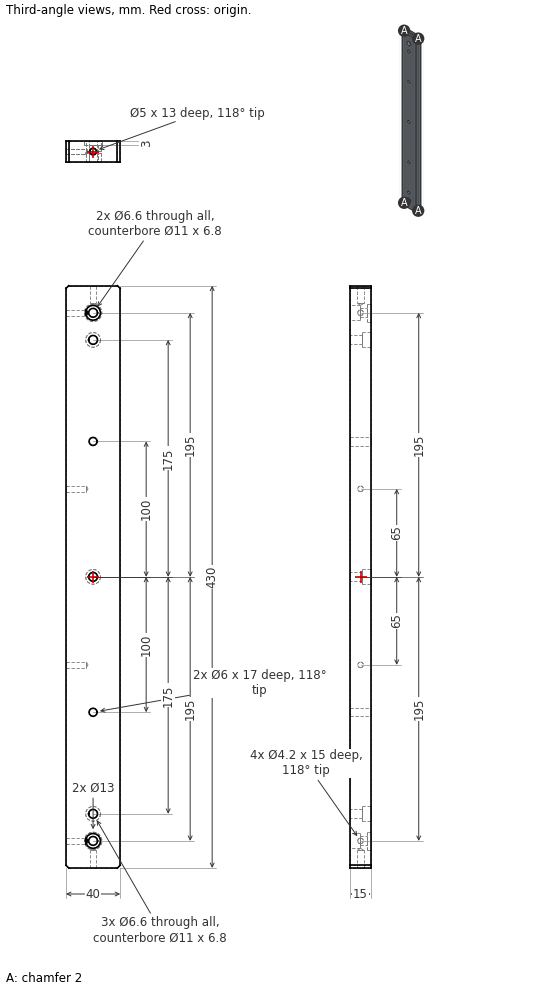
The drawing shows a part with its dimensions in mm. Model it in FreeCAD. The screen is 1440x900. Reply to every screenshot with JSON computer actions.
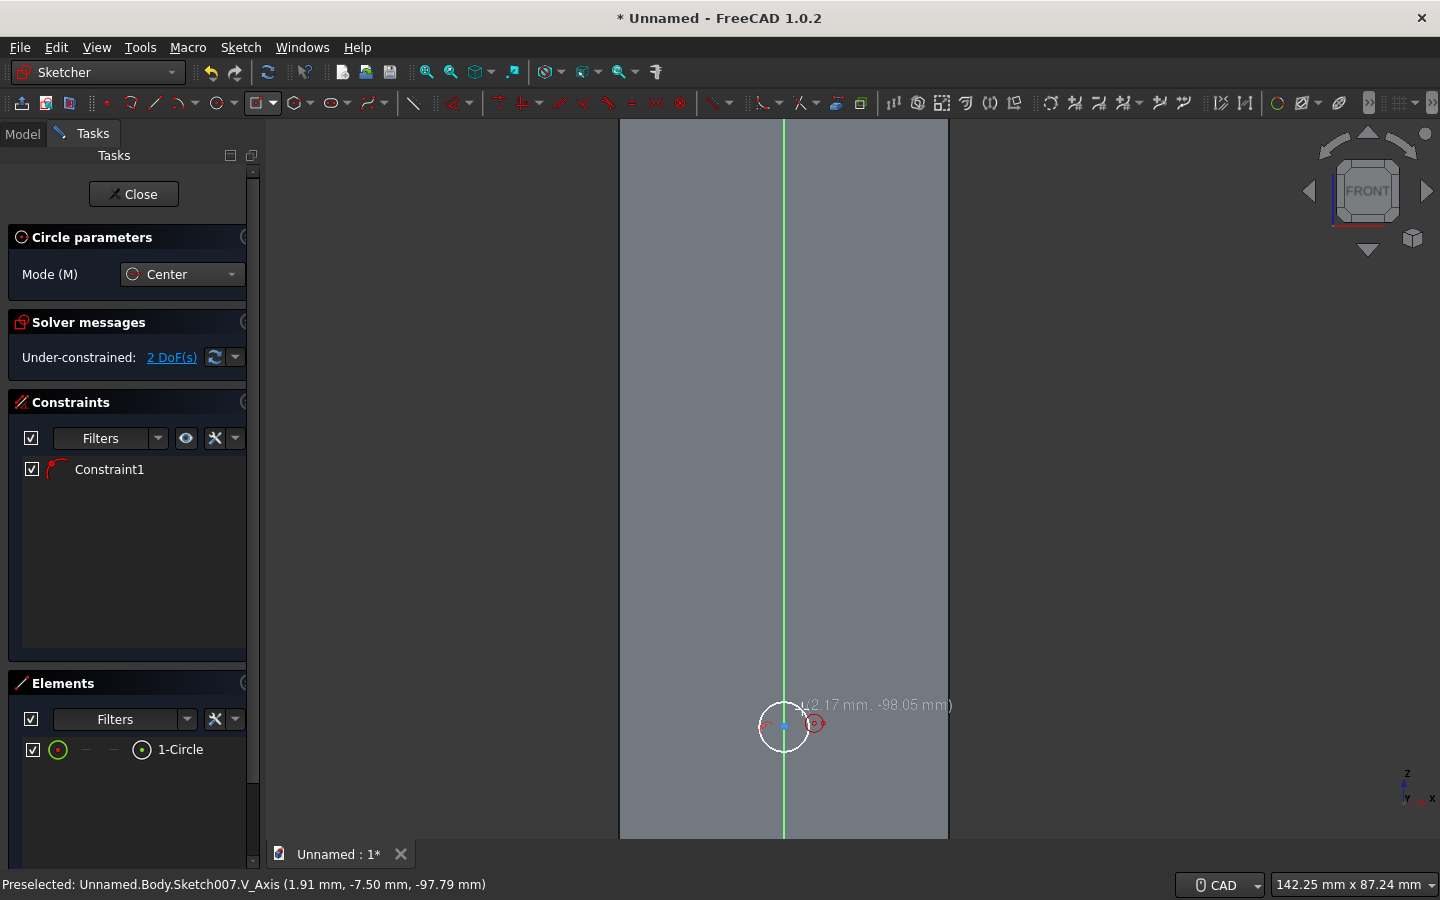
{"action": "scroll", "coordinate": [785, 728], "scroll_direction": "down", "scroll_amount": 6}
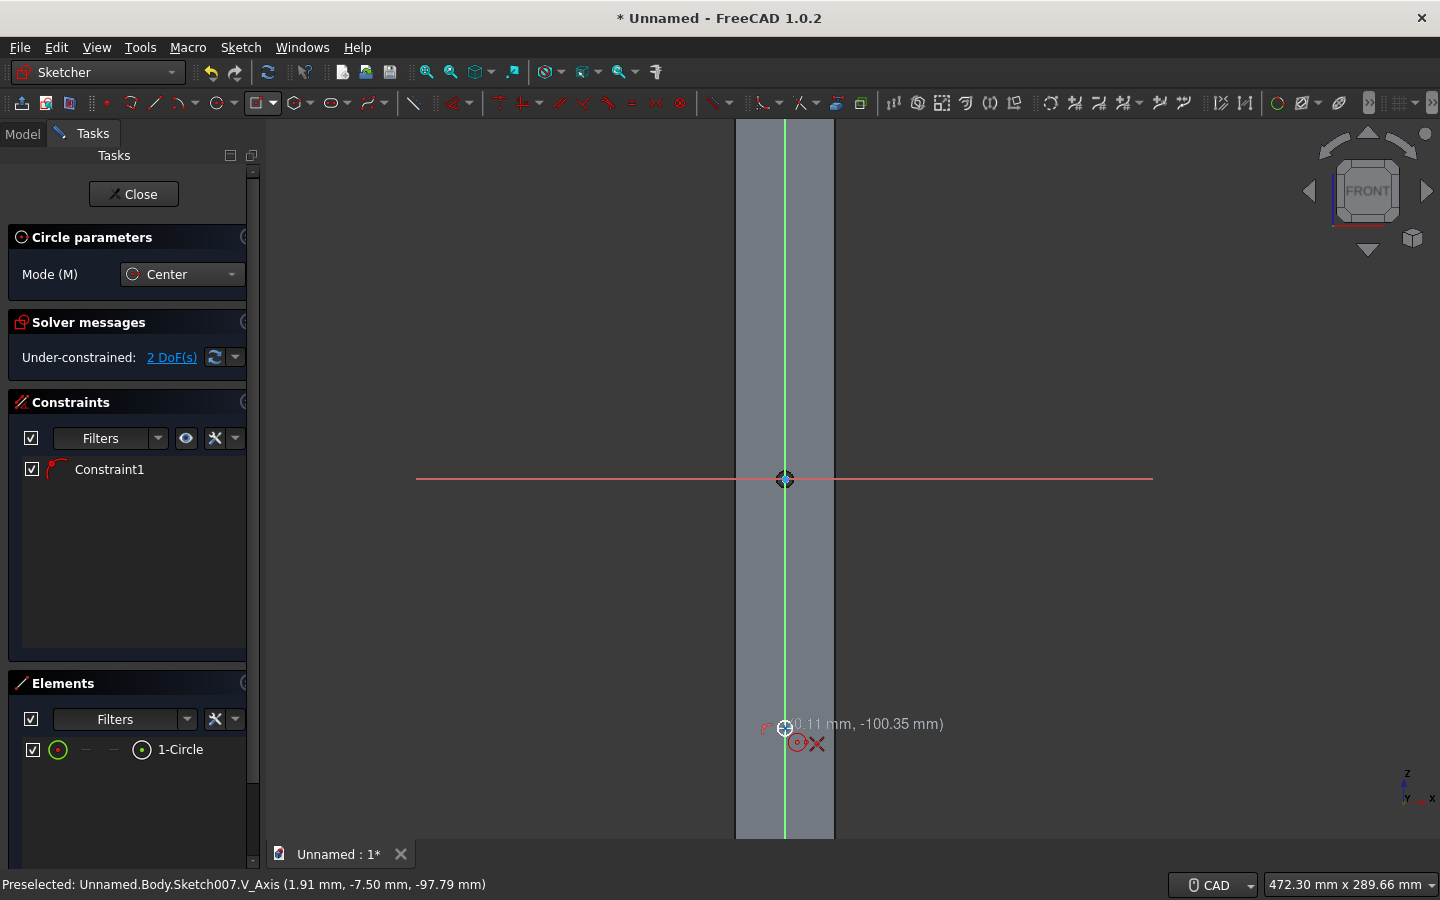
{"action": "scroll", "coordinate": [785, 231], "scroll_direction": "up", "scroll_amount": 6}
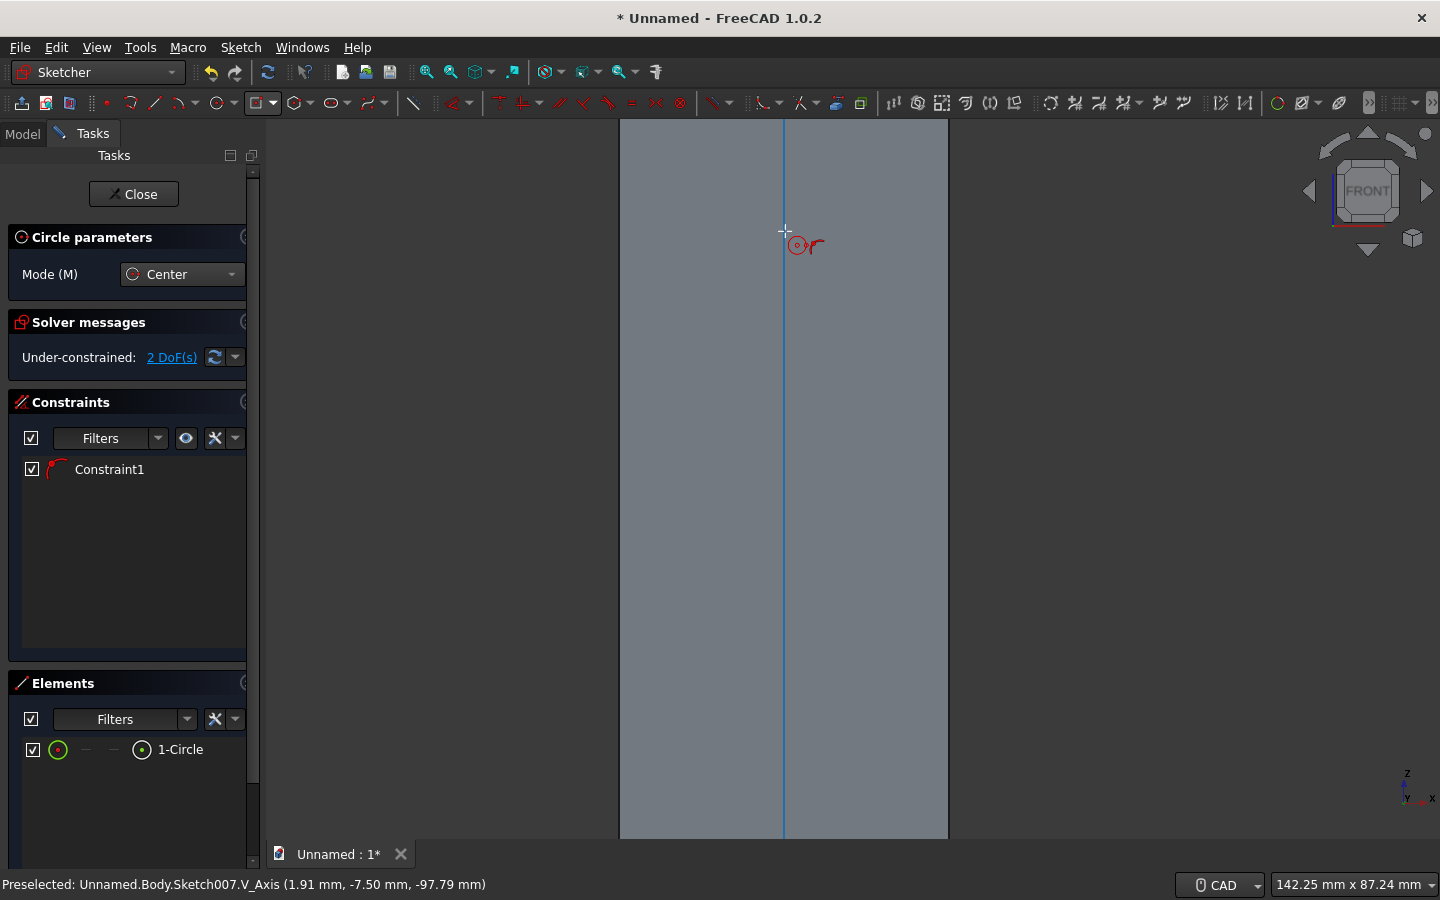
{"action": "left_click", "coordinate": [784, 230]}
{"action": "left_click", "coordinate": [802, 213]}
{"action": "key", "text": "Escape"}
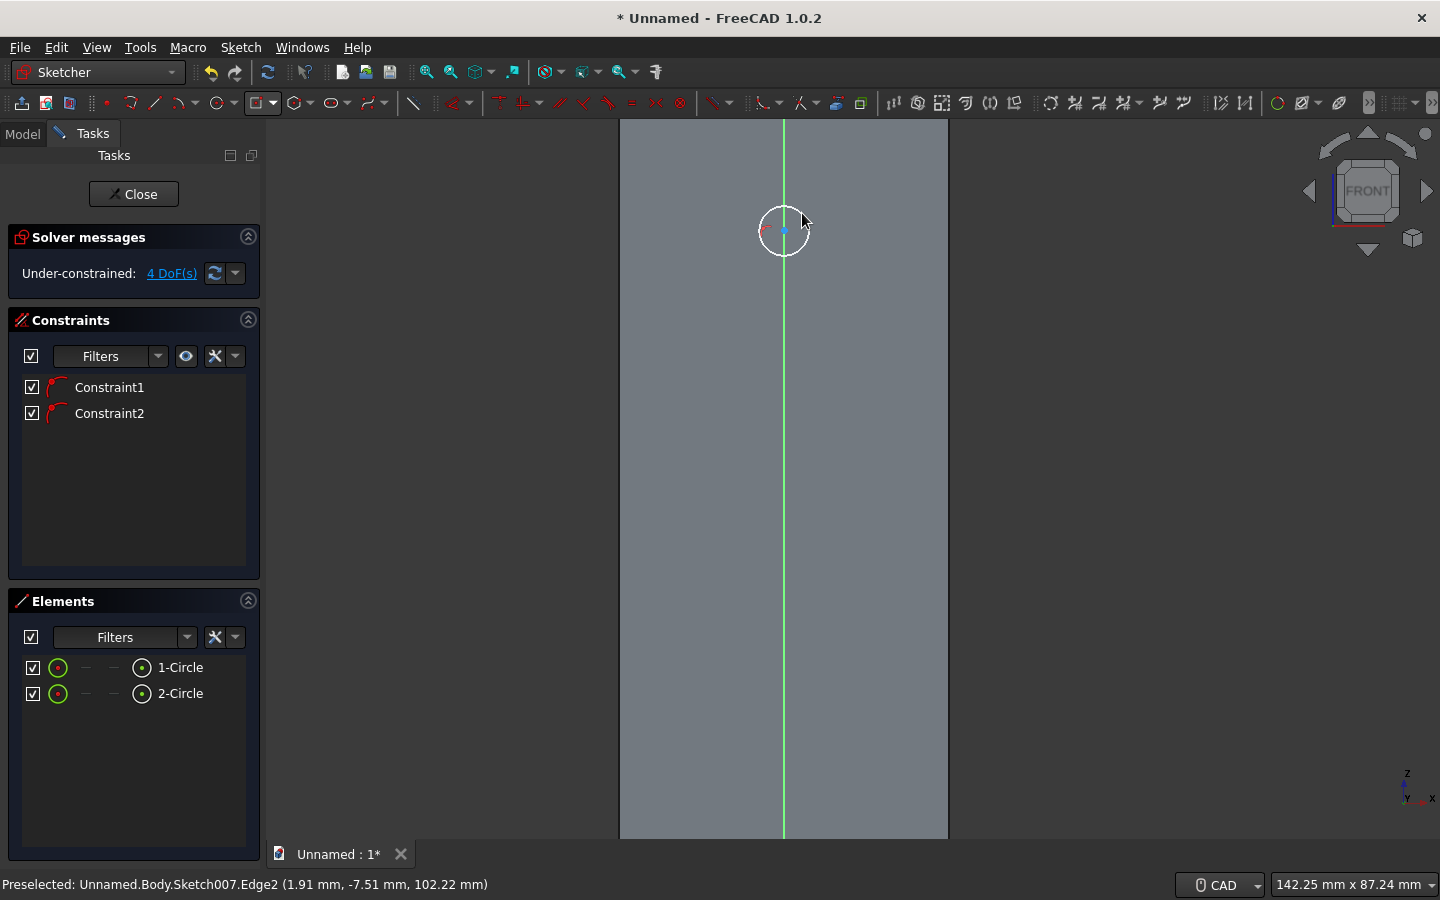
{"action": "scroll", "coordinate": [785, 231], "scroll_direction": "down", "scroll_amount": 6}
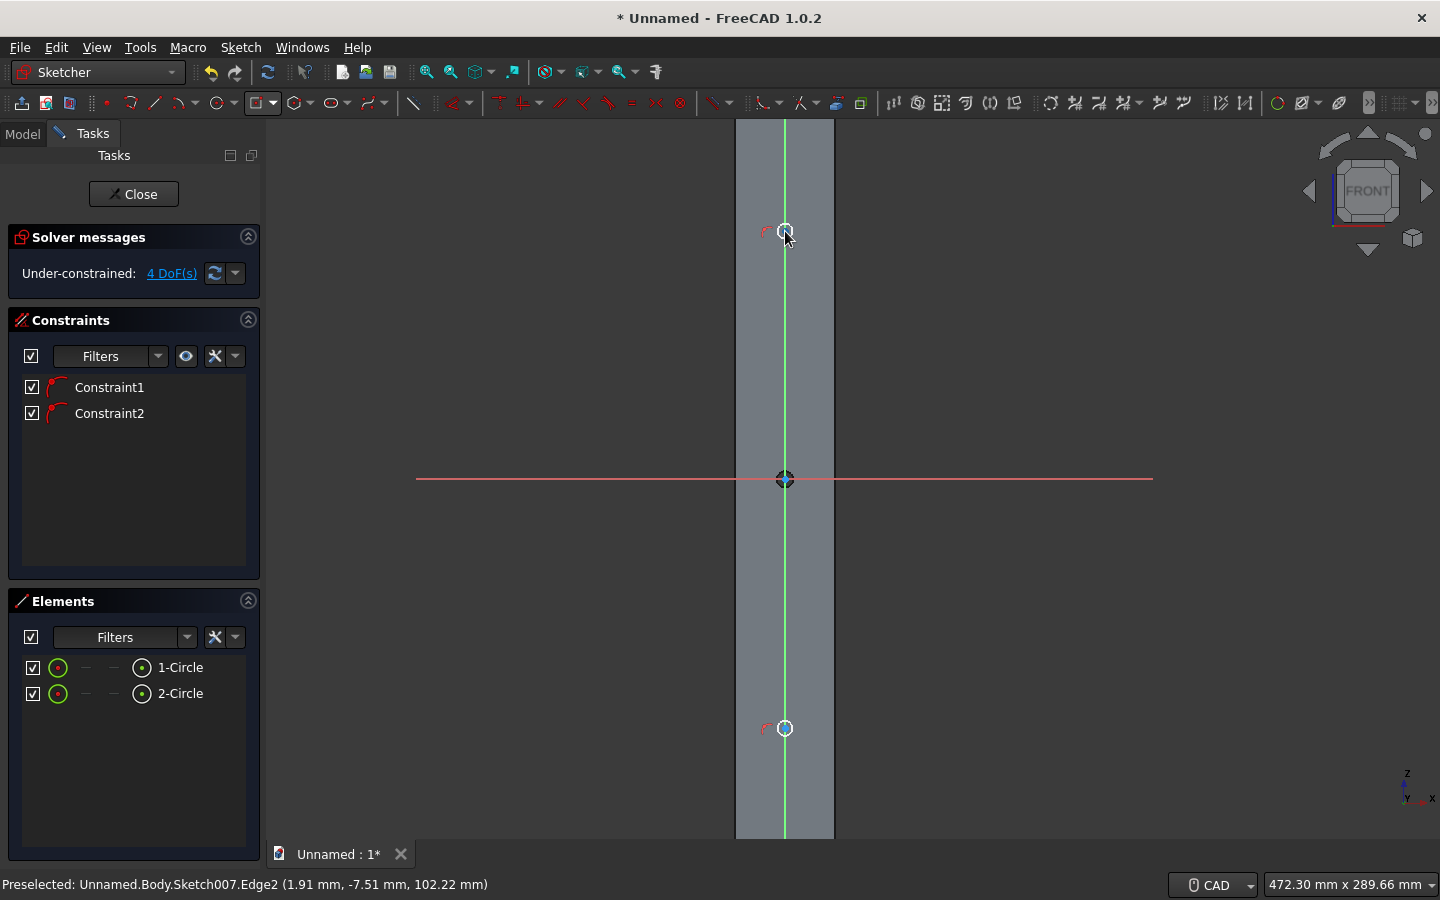
{"action": "scroll", "coordinate": [790, 723], "scroll_direction": "up", "scroll_amount": 5}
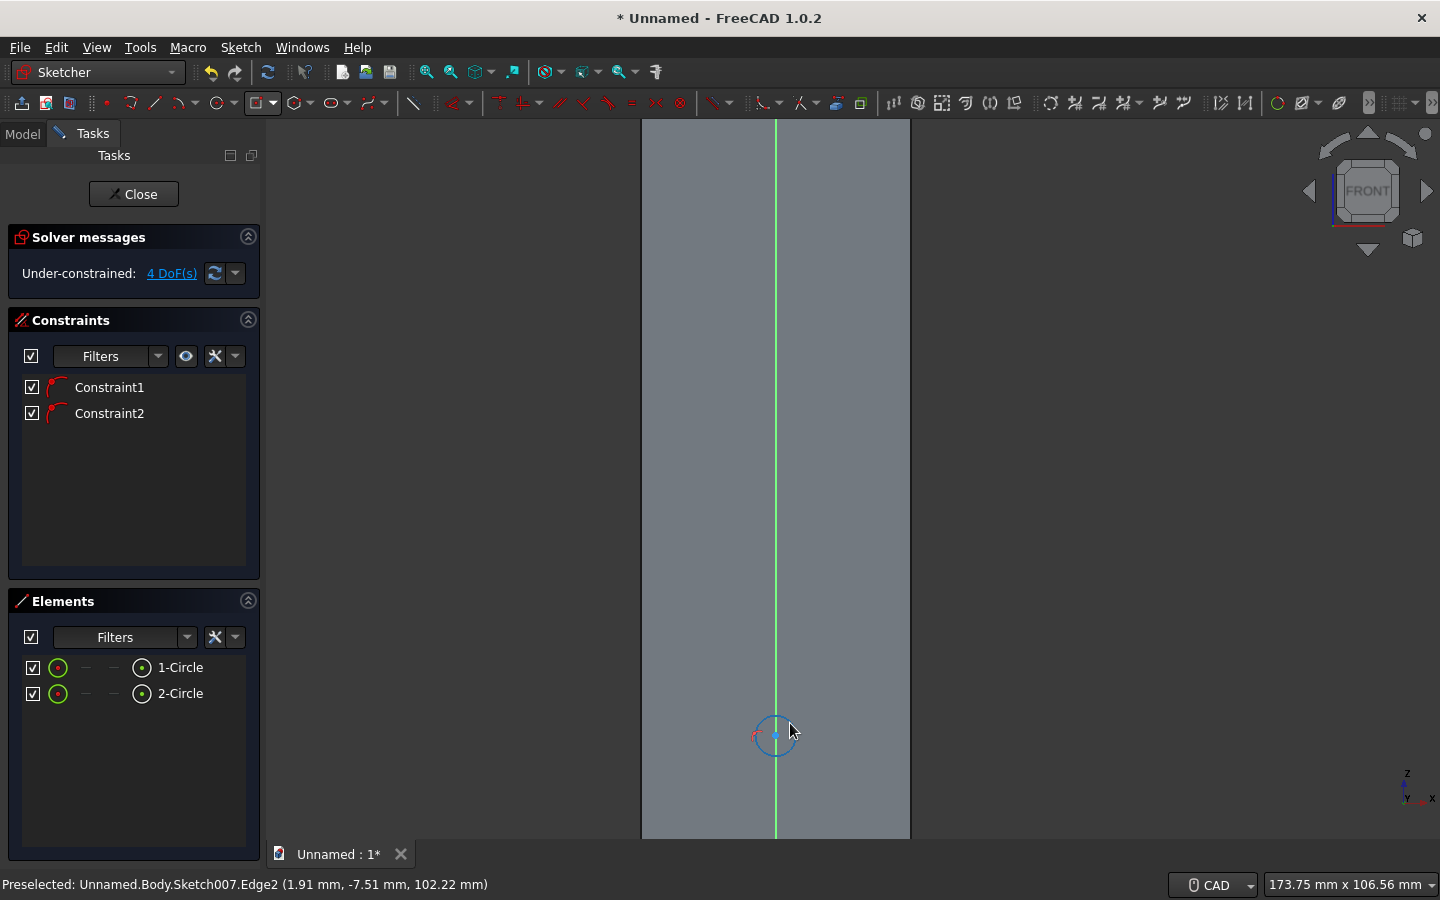
{"action": "left_click", "coordinate": [790, 722]}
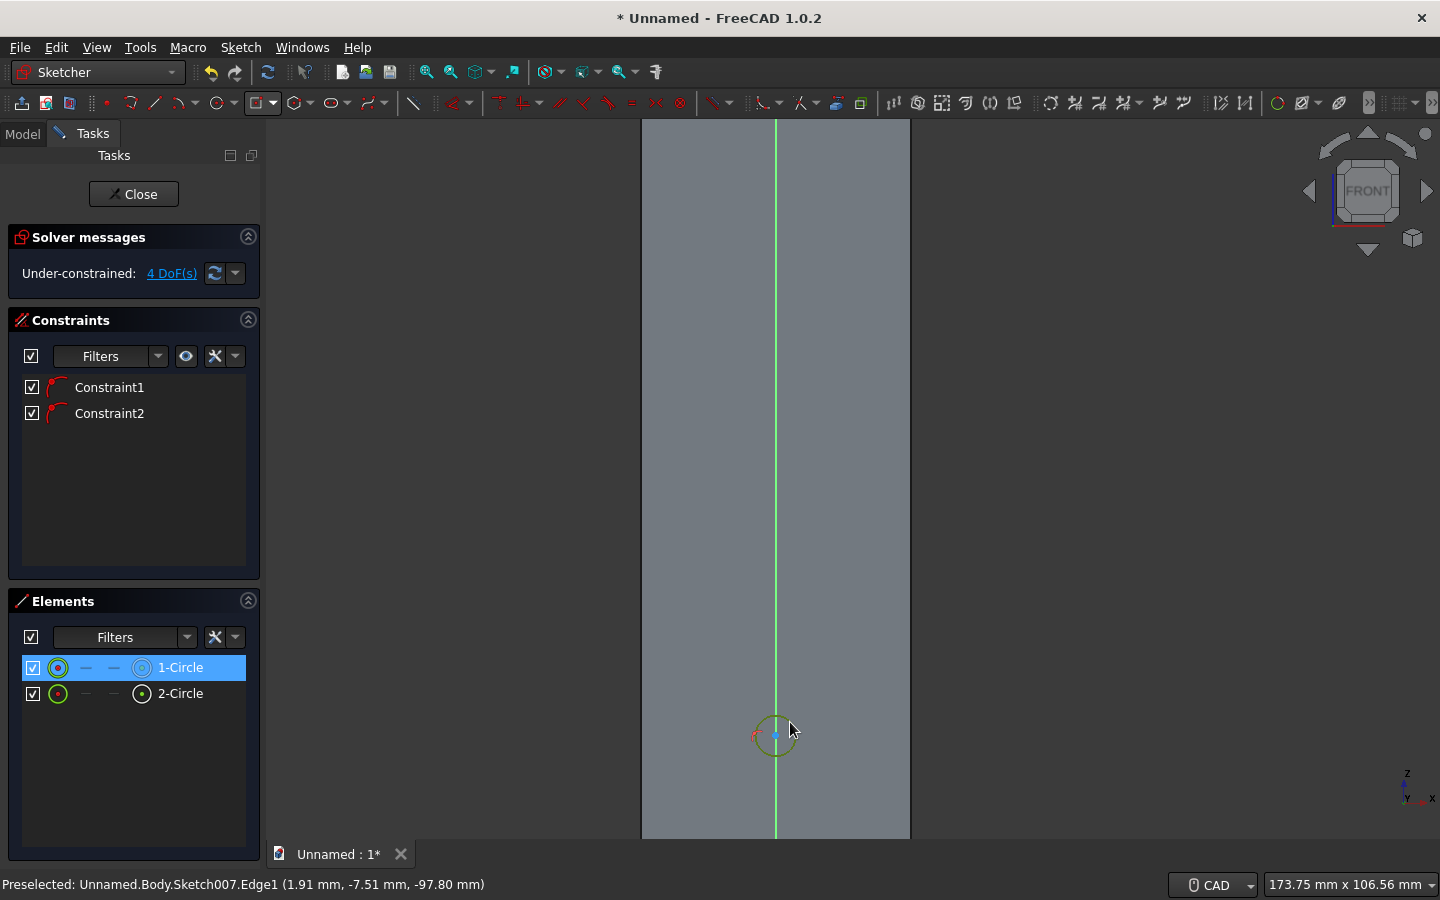
{"action": "scroll", "coordinate": [790, 723], "scroll_direction": "down", "scroll_amount": 5}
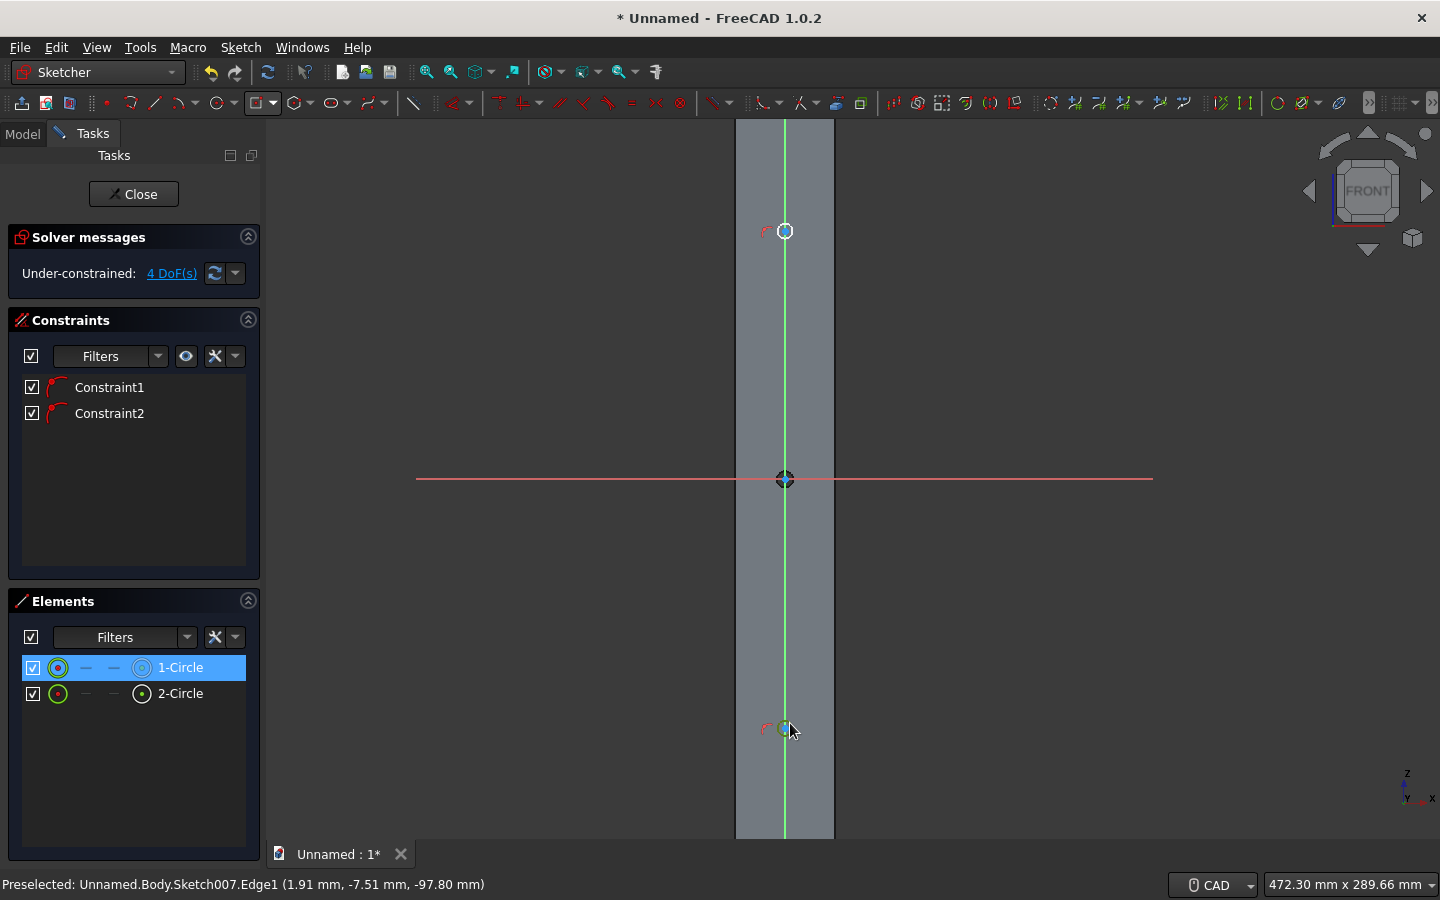
{"action": "scroll", "coordinate": [790, 226], "scroll_direction": "up", "scroll_amount": 5}